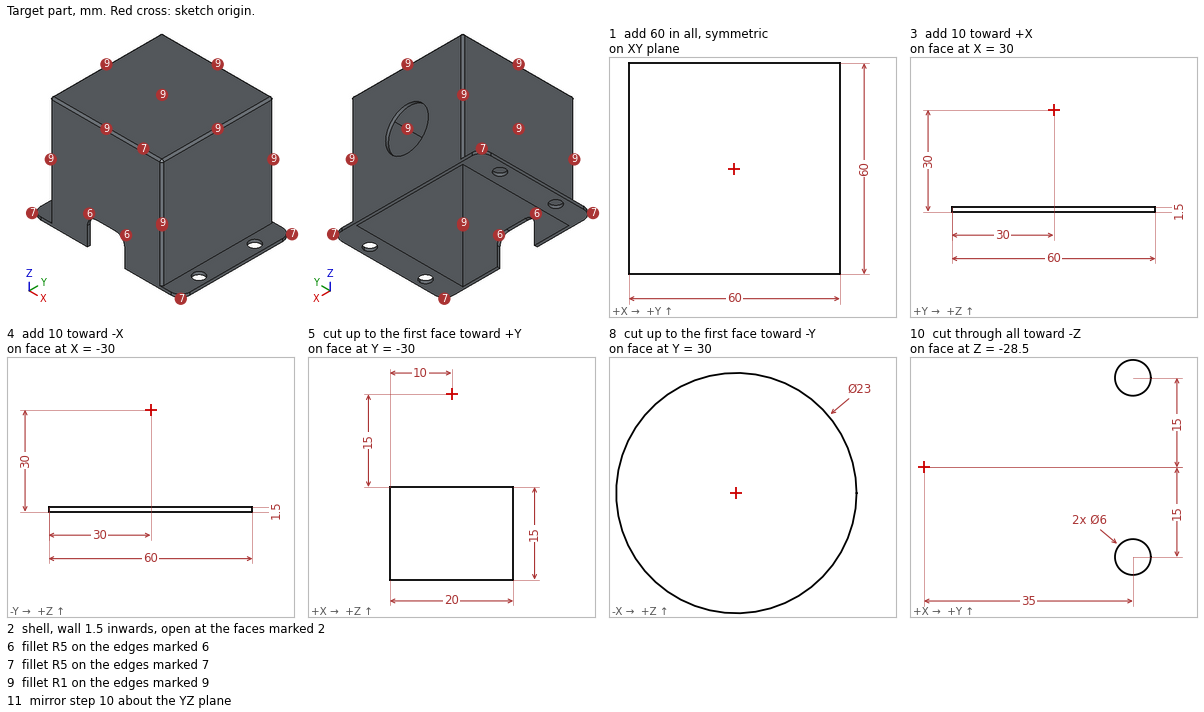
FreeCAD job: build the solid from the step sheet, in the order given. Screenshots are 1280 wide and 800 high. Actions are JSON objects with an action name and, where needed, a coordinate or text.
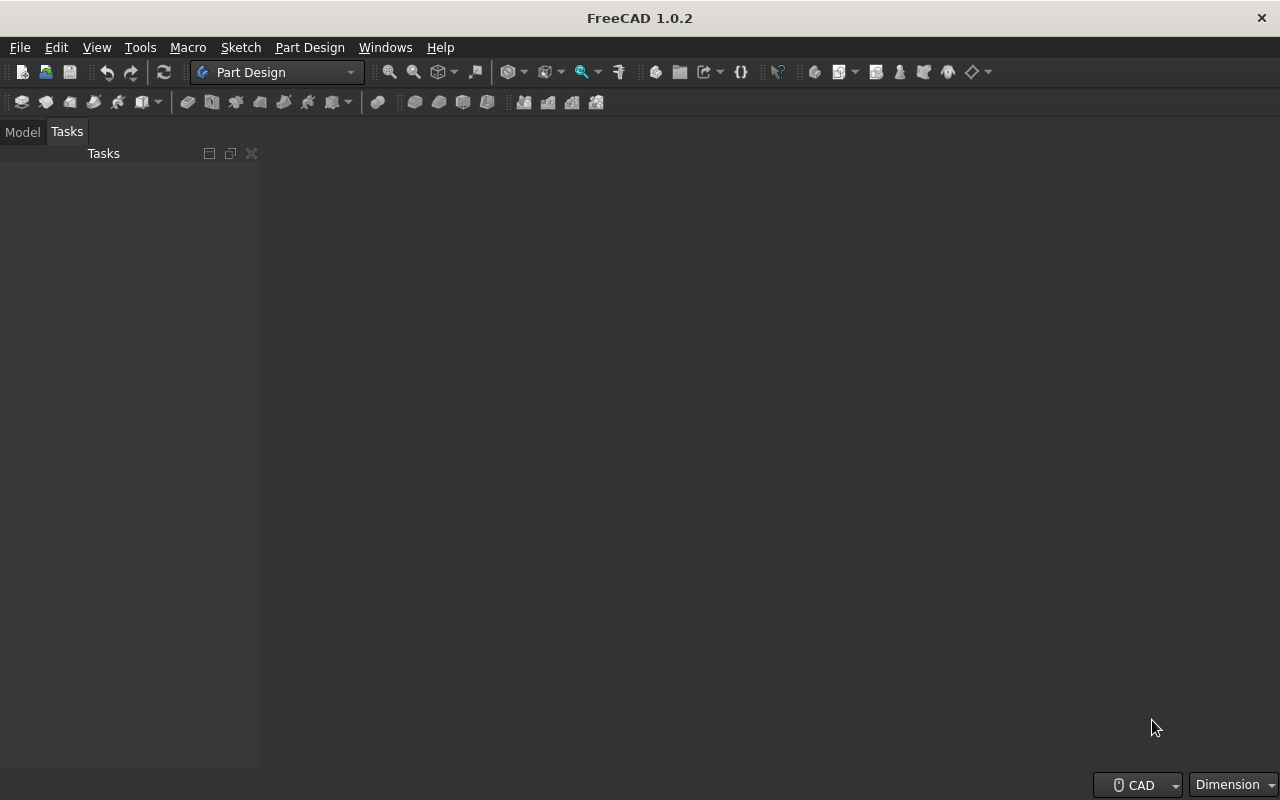
{"action": "left_click", "coordinate": [22, 72]}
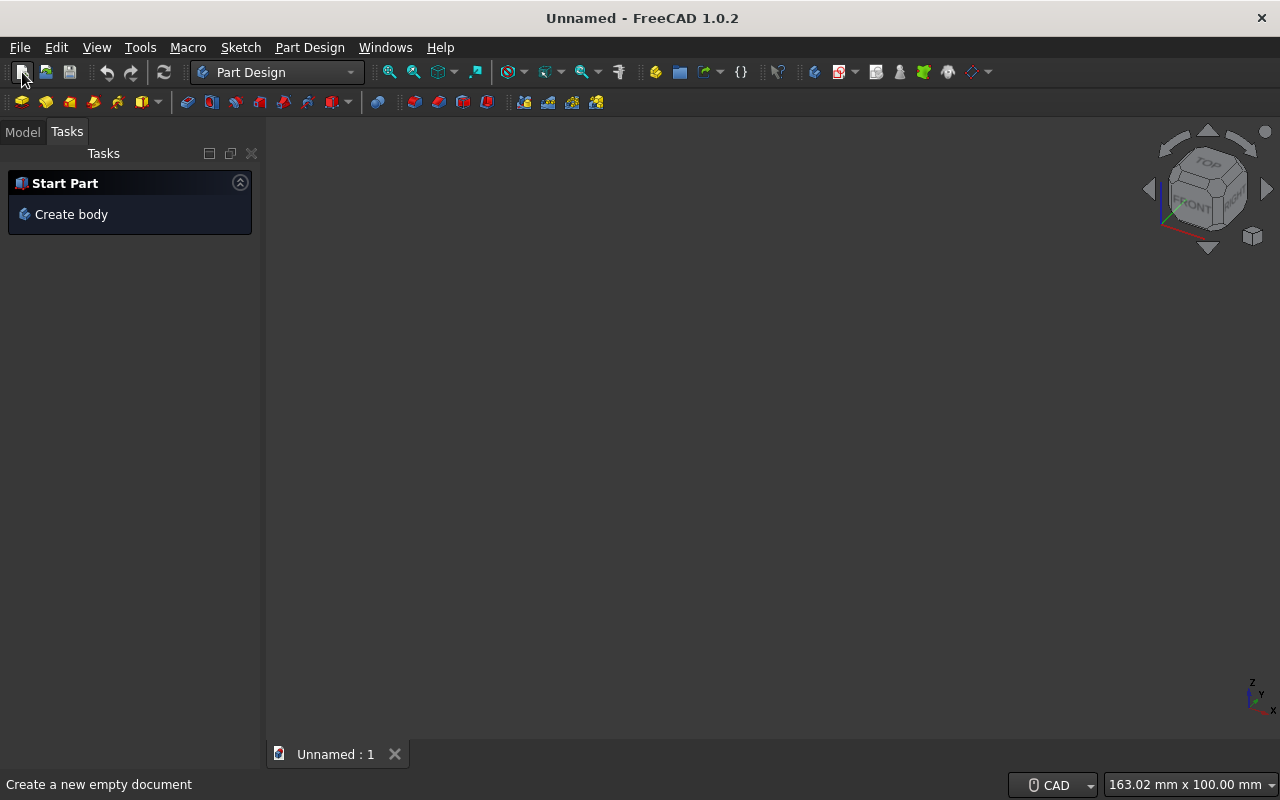
{"action": "left_click", "coordinate": [840, 72]}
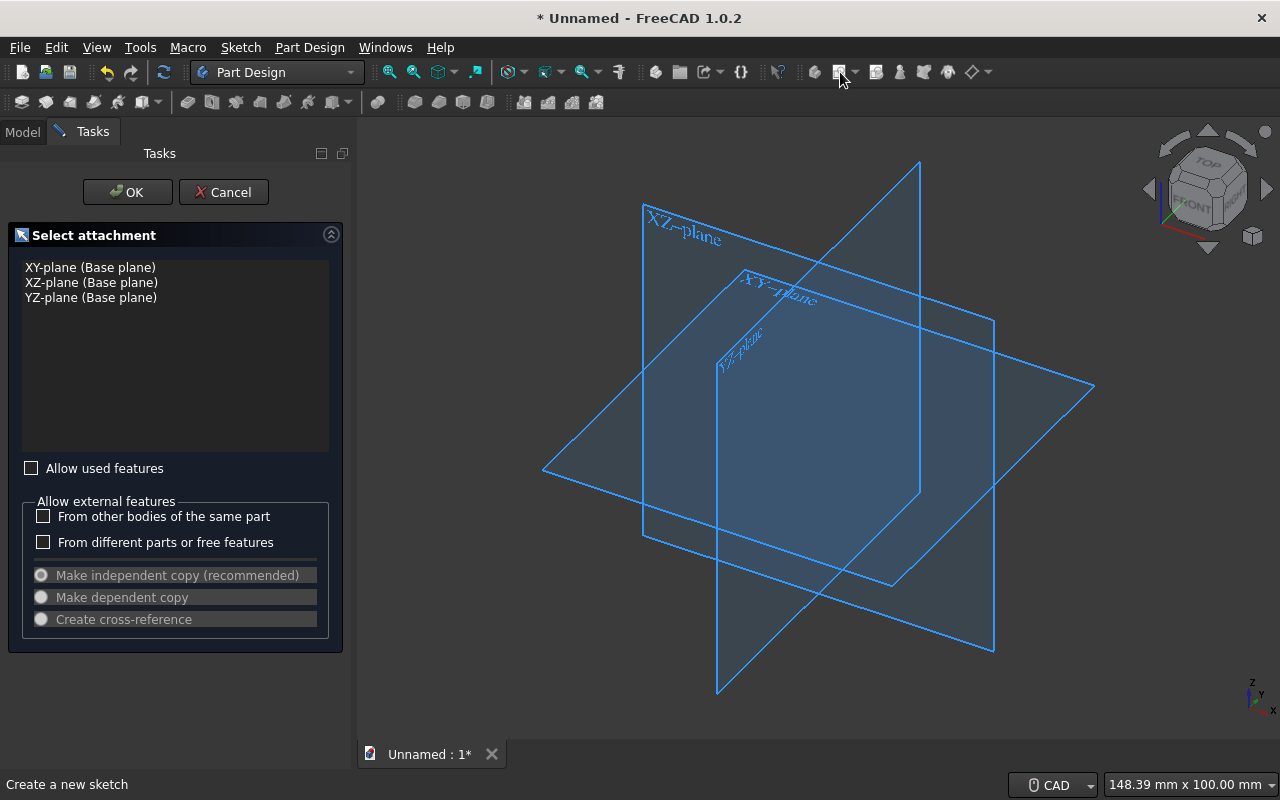
{"action": "left_click", "coordinate": [82, 268]}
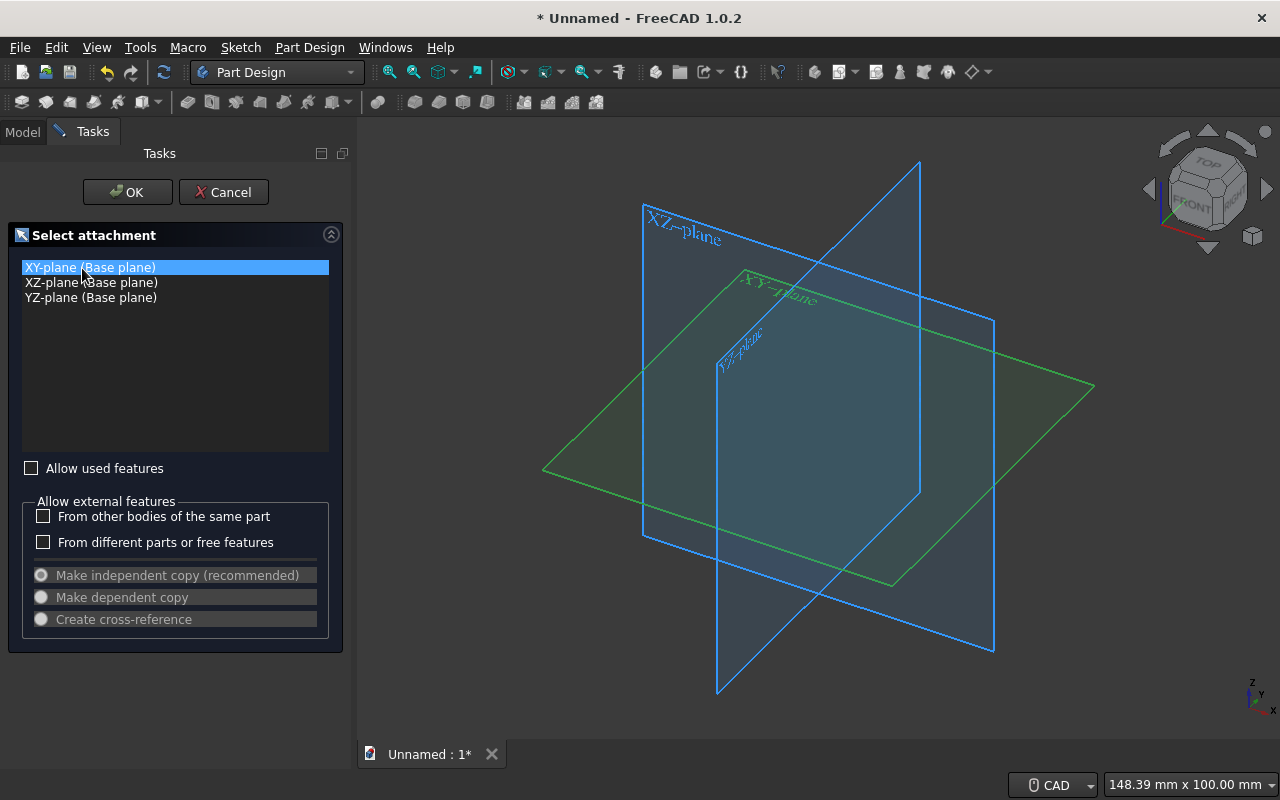
{"action": "left_click", "coordinate": [128, 192]}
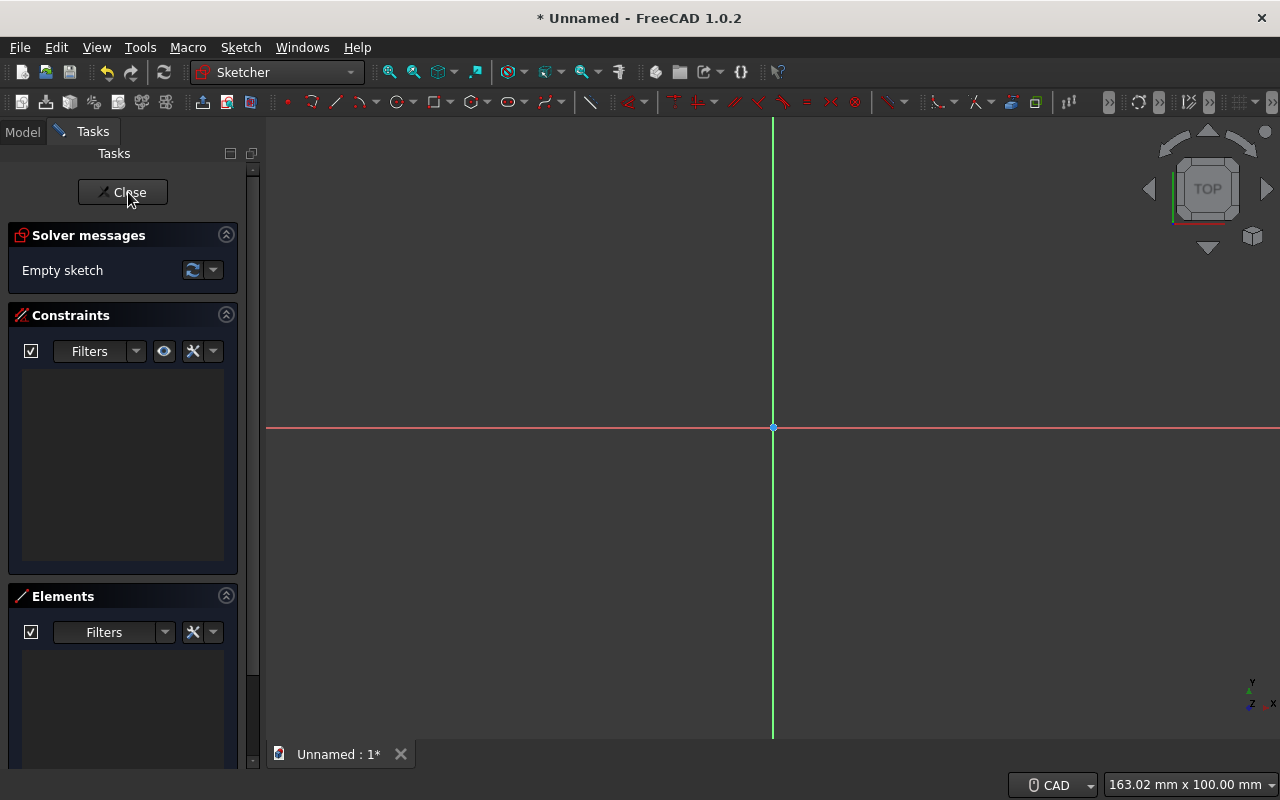
{"action": "key", "text": "g v"}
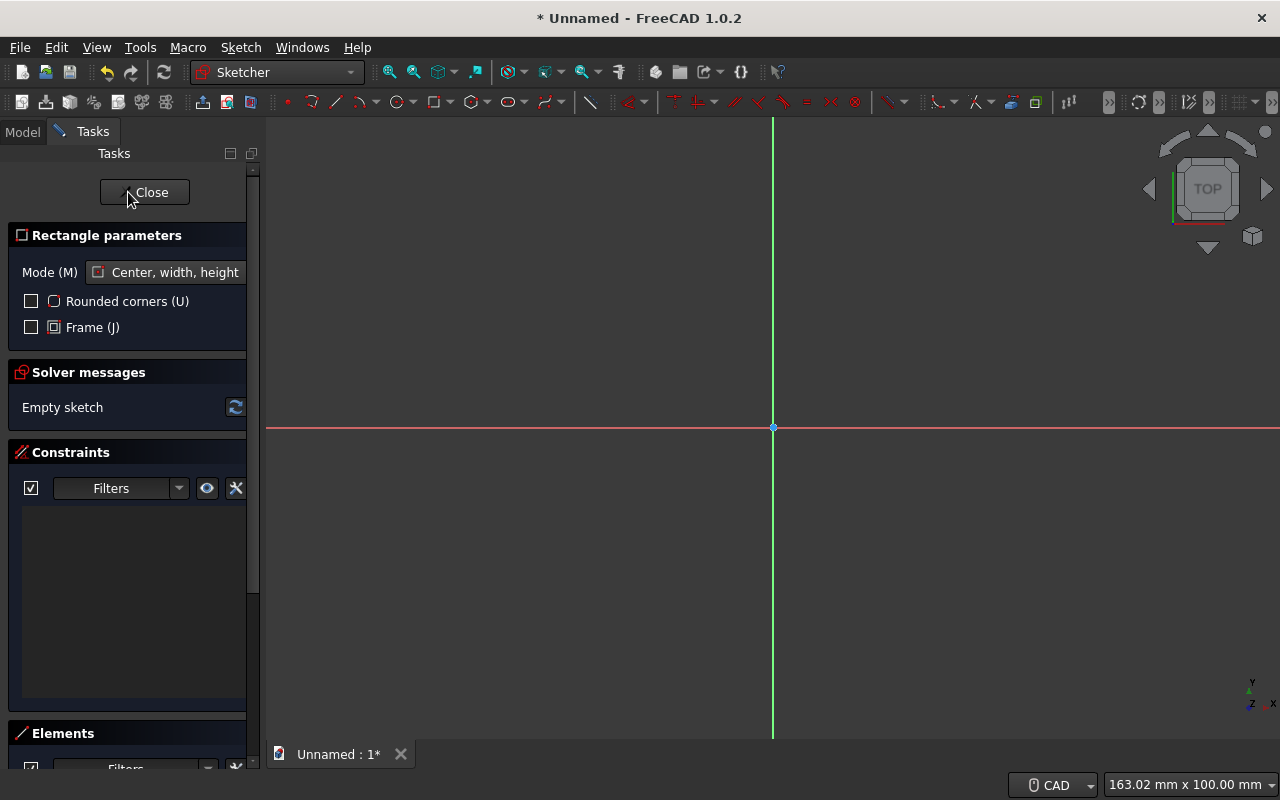
{"action": "left_click", "coordinate": [773, 428]}
{"action": "mouse_move", "coordinate": [960, 241]}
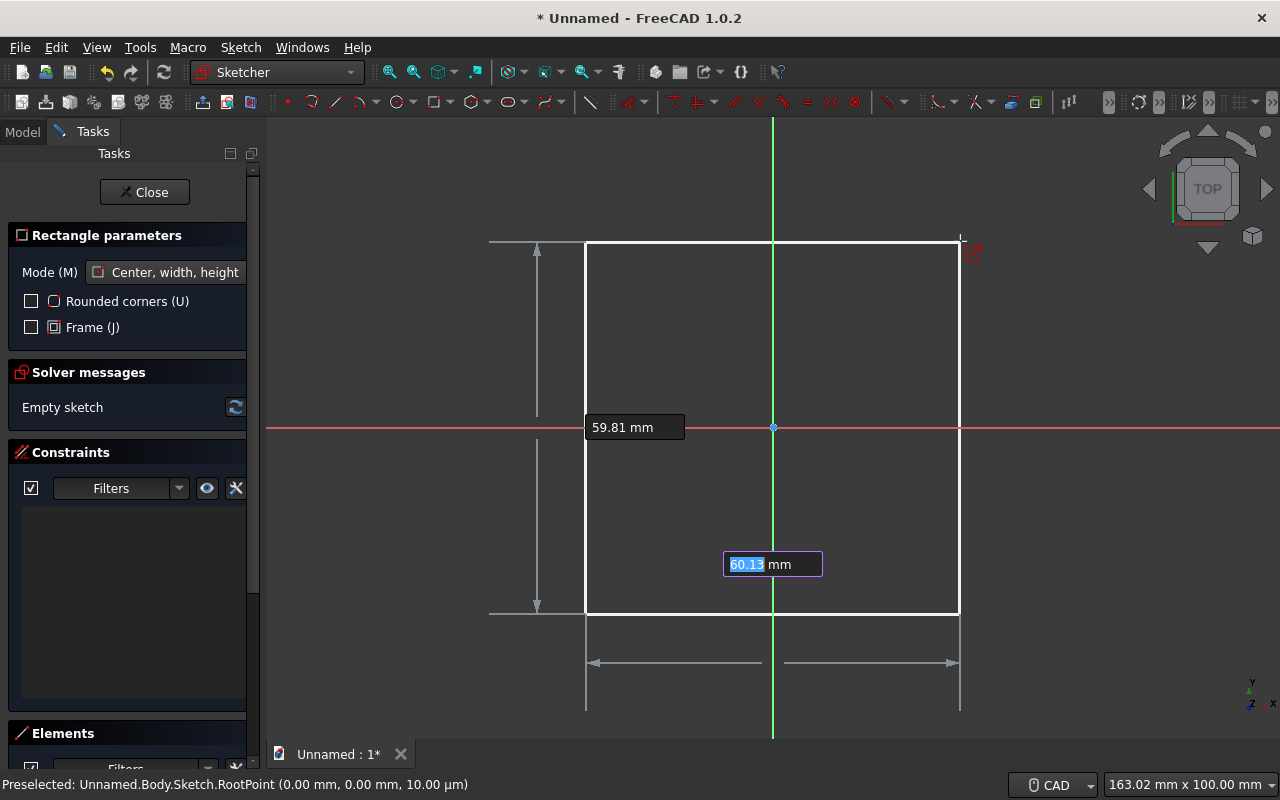
{"action": "type", "text": "60"}
{"action": "key", "text": "Tab"}
{"action": "type", "text": "60"}
{"action": "key", "text": "Return"}
{"action": "key", "text": "Escape"}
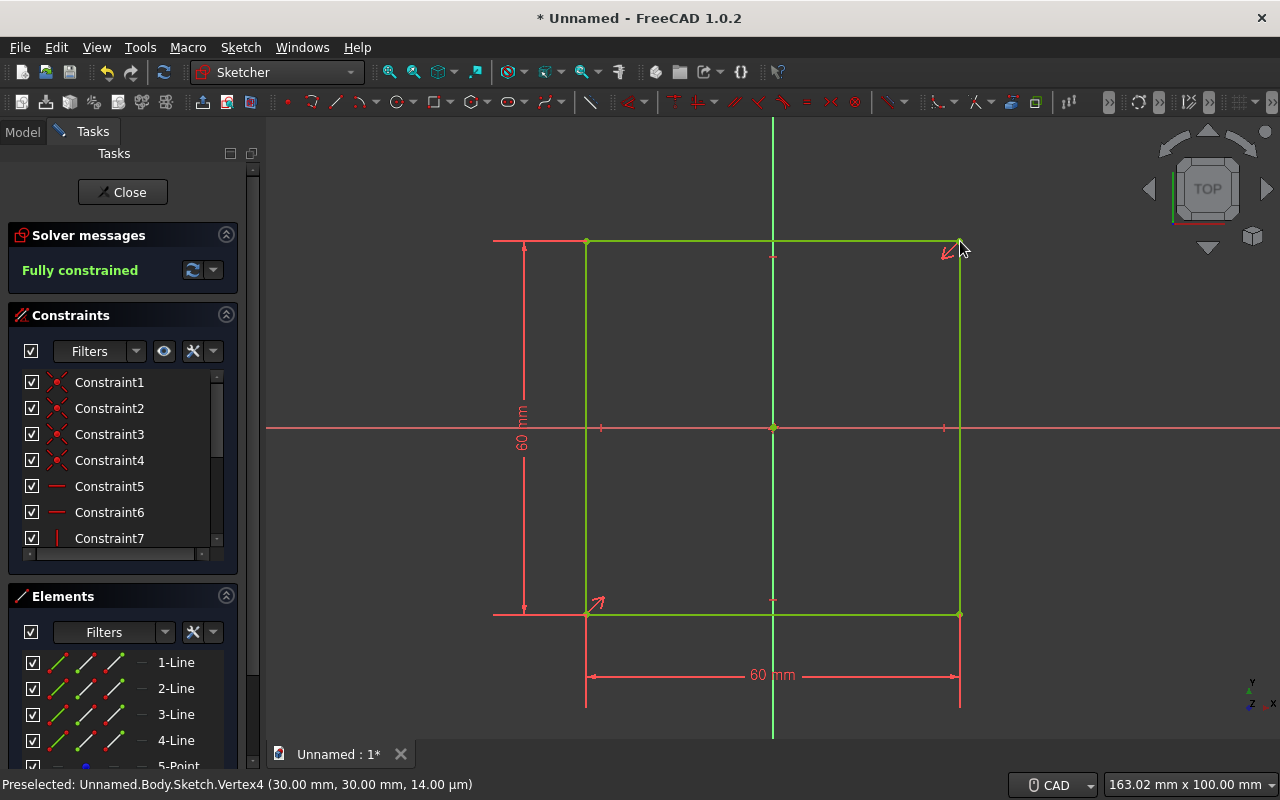
{"action": "left_click", "coordinate": [123, 192]}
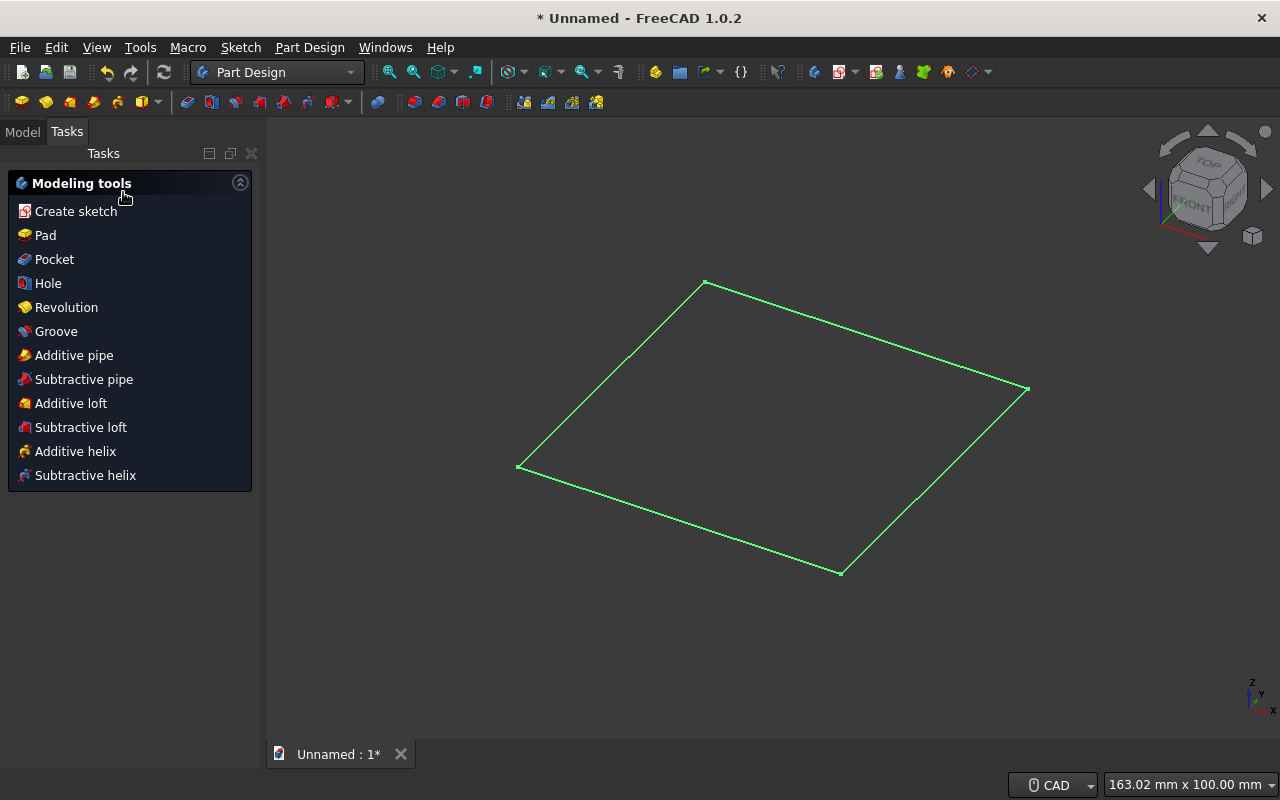
{"action": "left_click", "coordinate": [22, 102]}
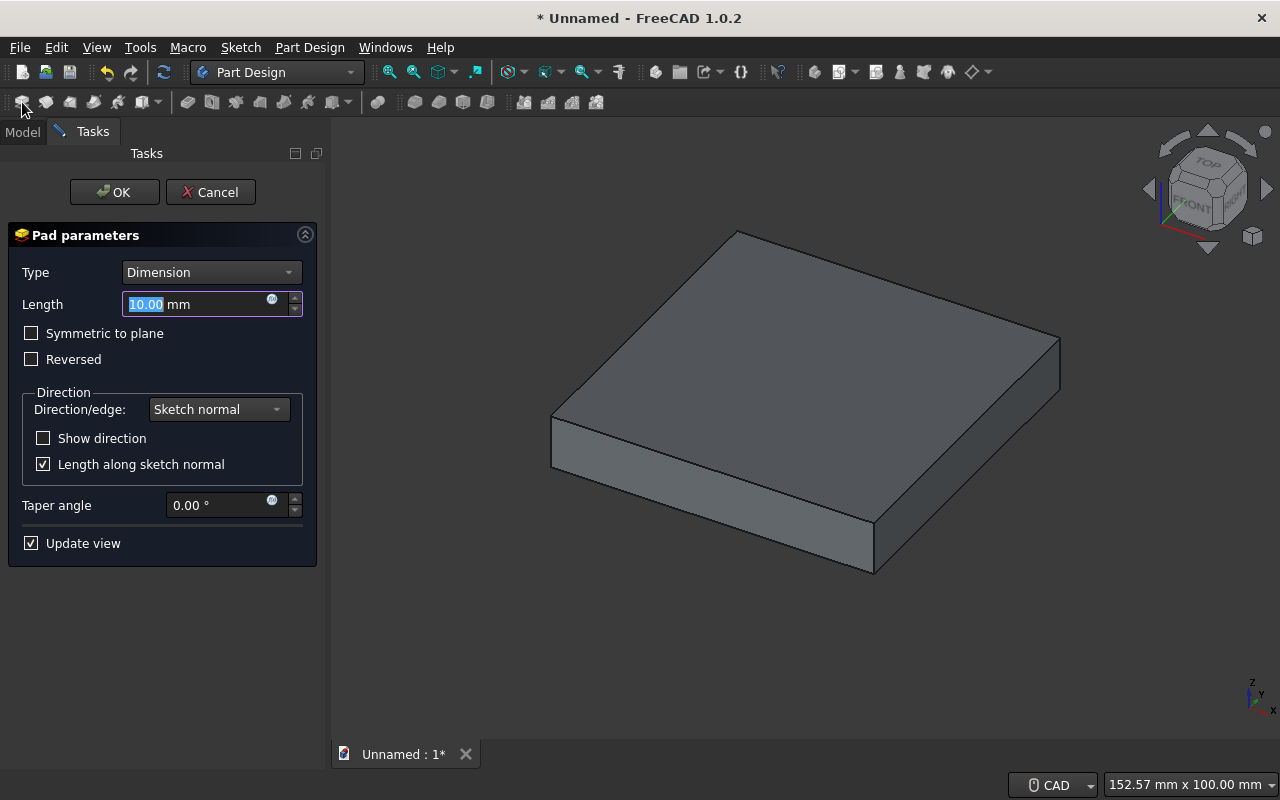
{"action": "type", "text": "60"}
{"action": "key", "text": "Tab"}